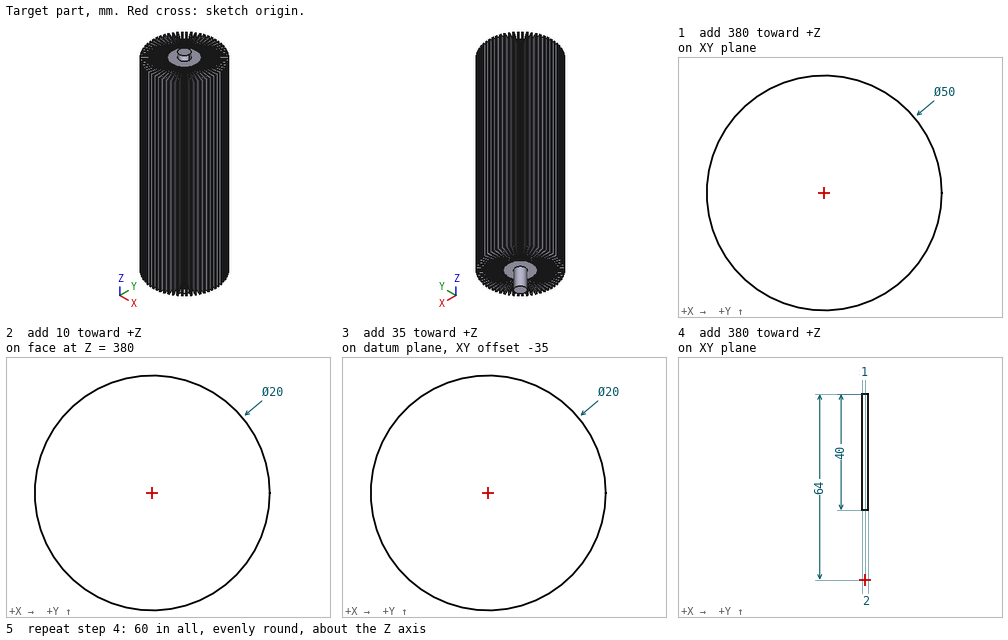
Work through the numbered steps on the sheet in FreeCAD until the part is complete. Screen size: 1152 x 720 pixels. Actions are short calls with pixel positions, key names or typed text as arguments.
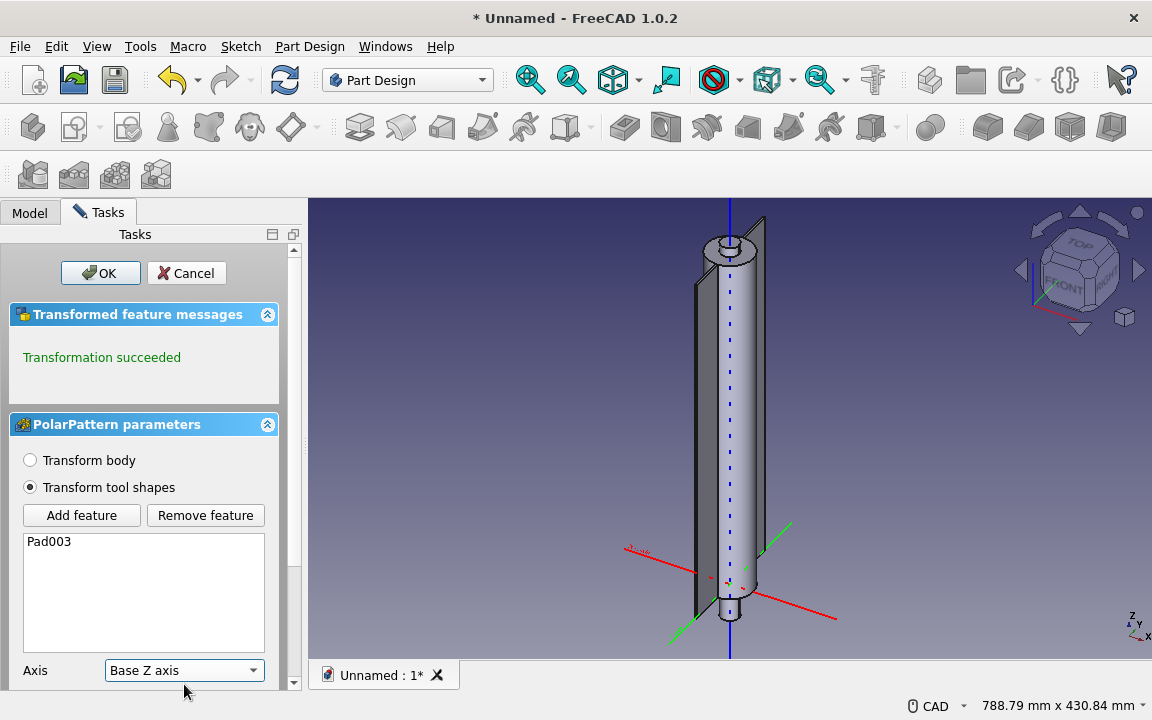
scroll(294, 467, down, 3)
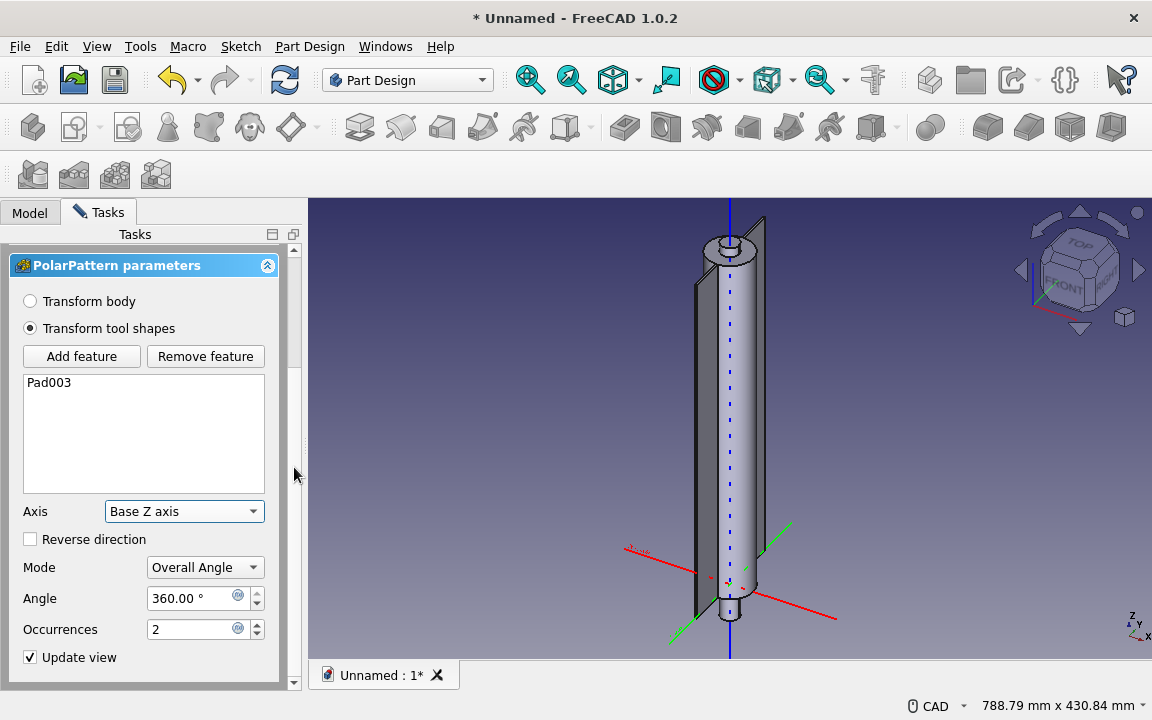
triple_click(199, 630)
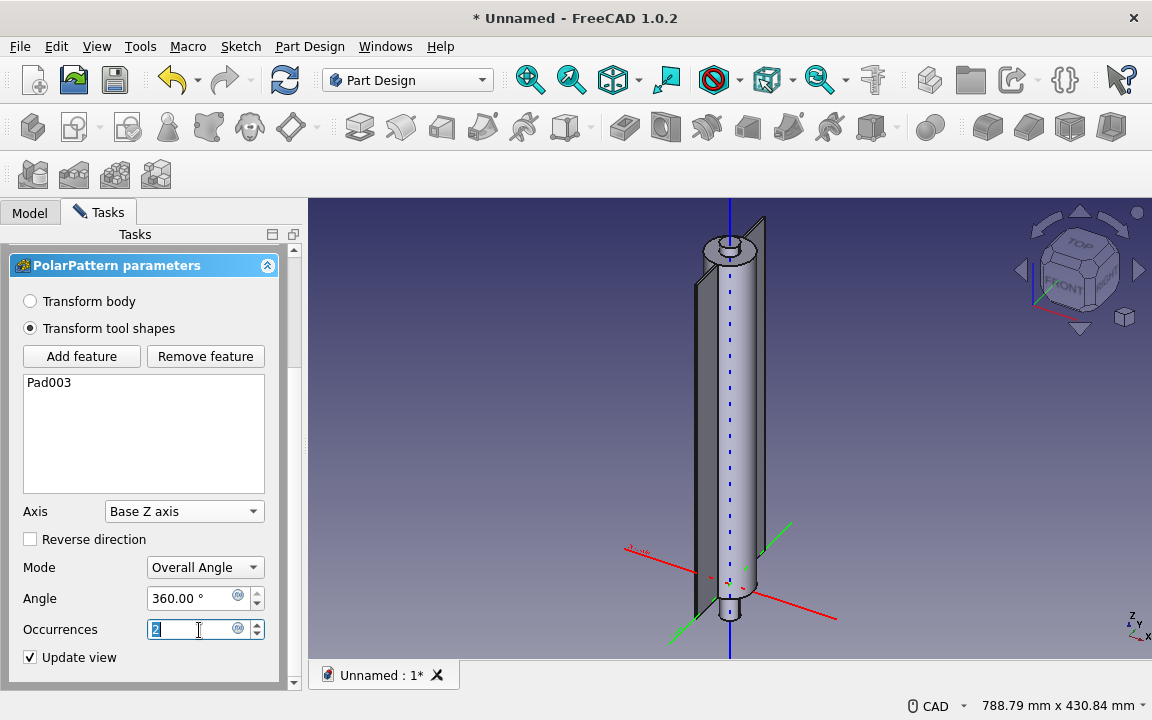
text(60)
key(Tab)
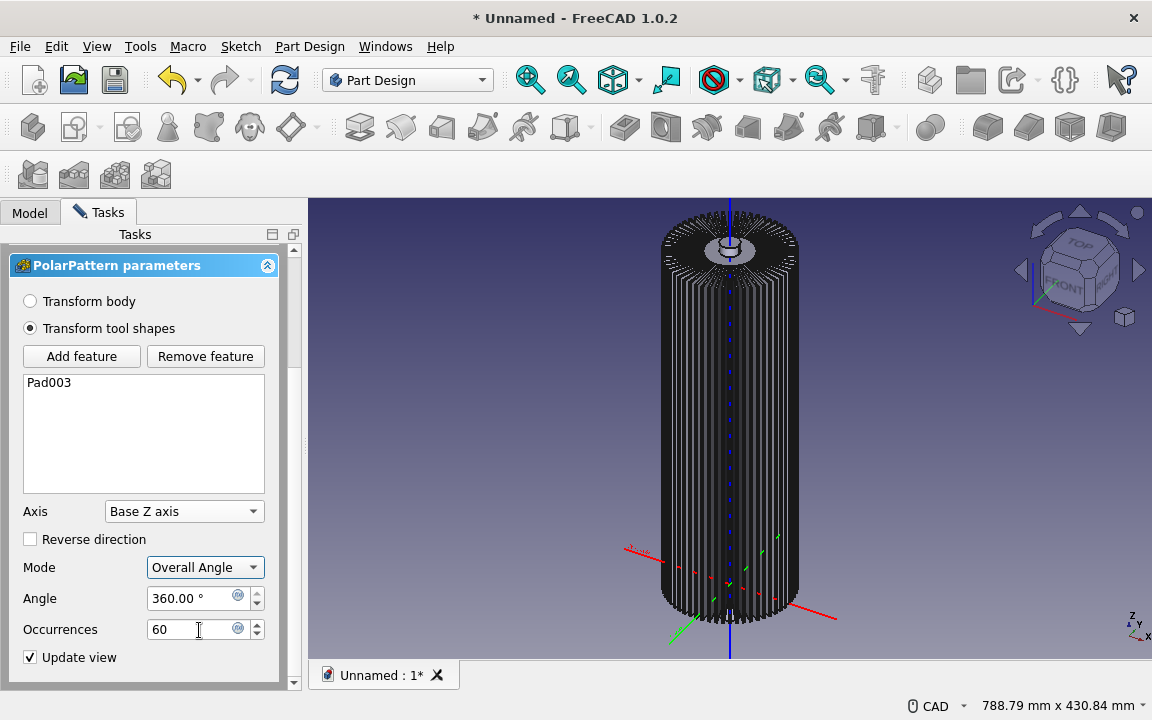
scroll(294, 467, up, 4)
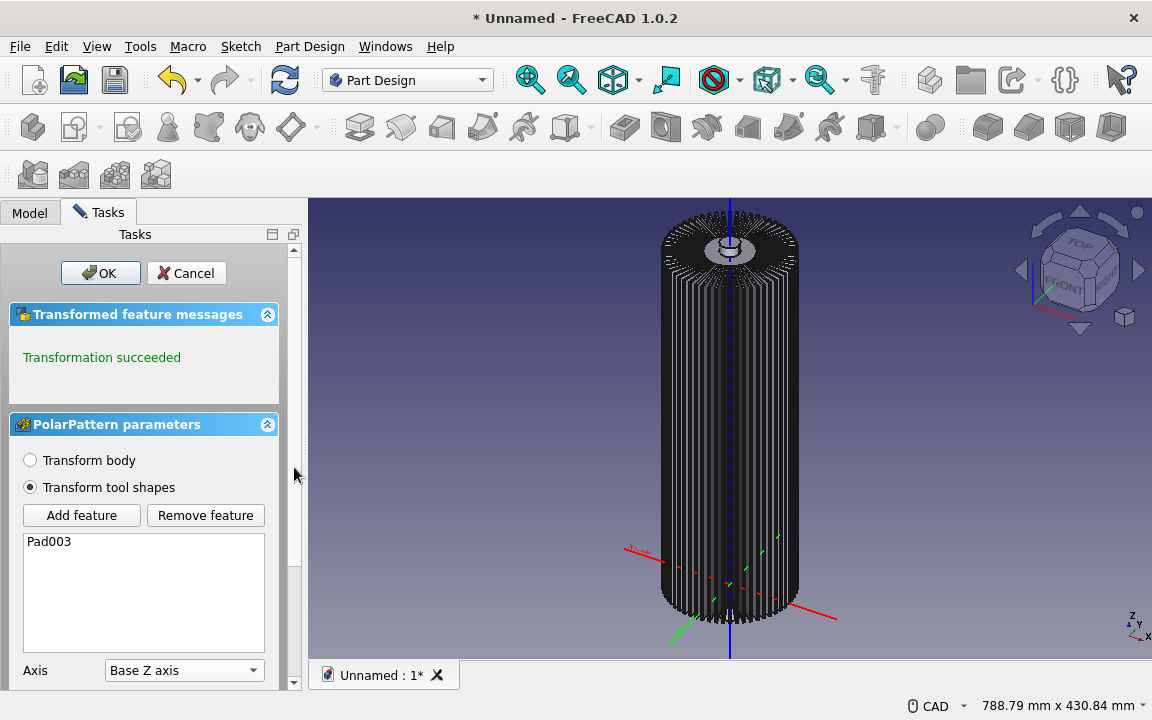
click(101, 273)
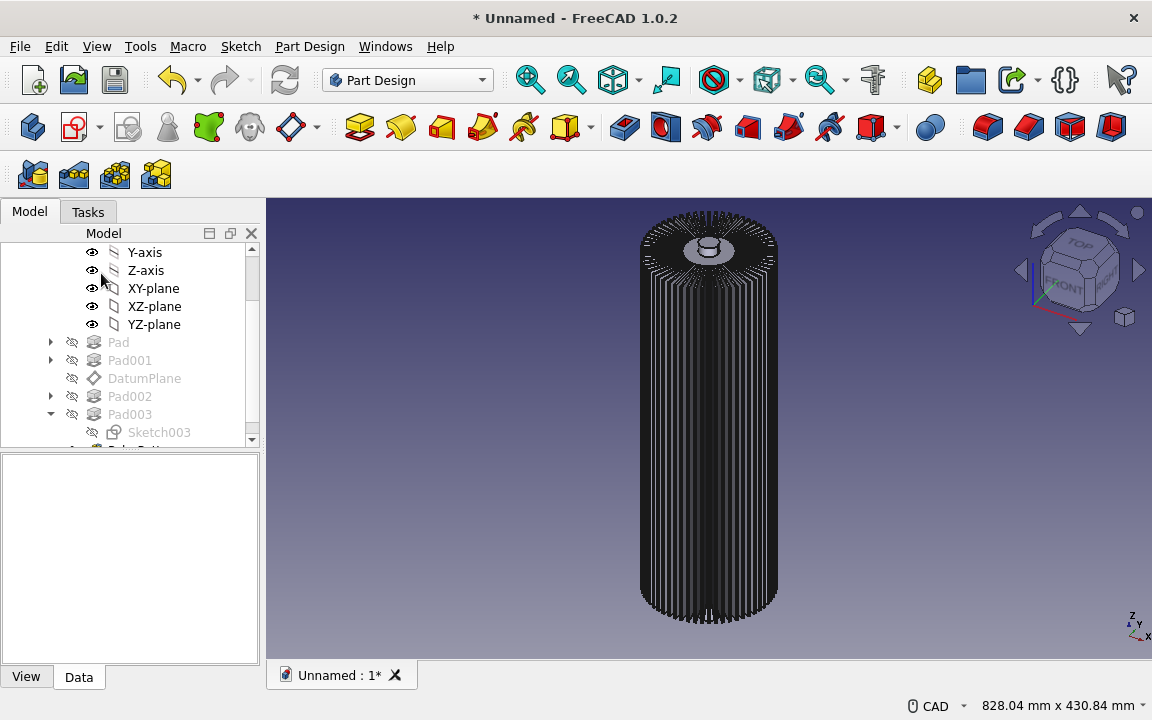
key(0)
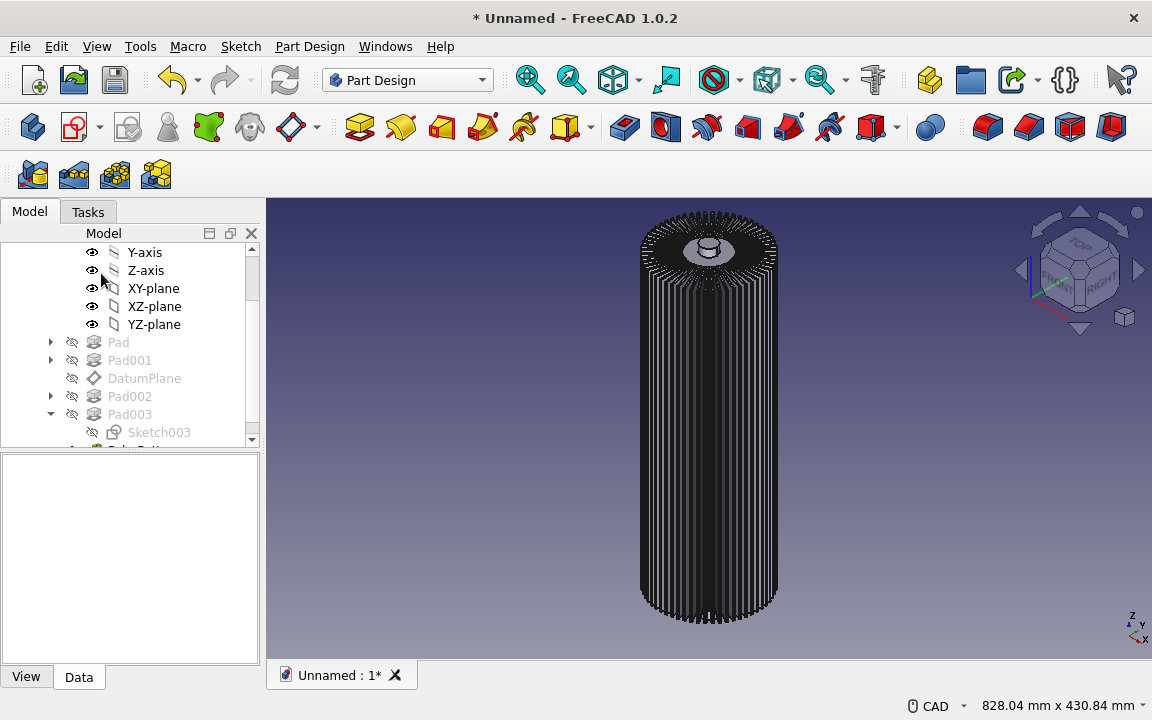
click(531, 80)